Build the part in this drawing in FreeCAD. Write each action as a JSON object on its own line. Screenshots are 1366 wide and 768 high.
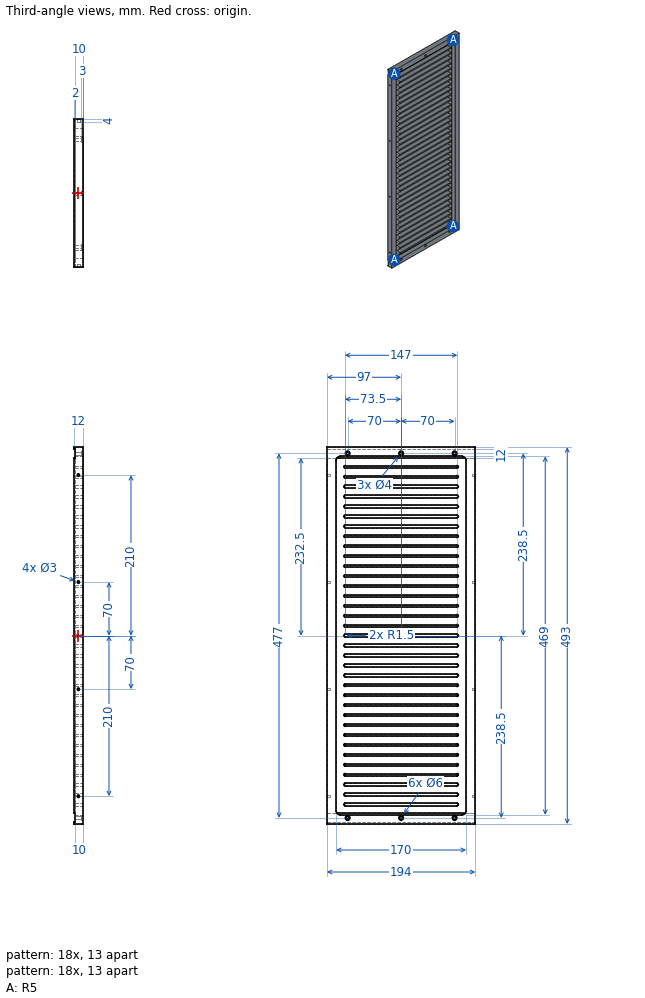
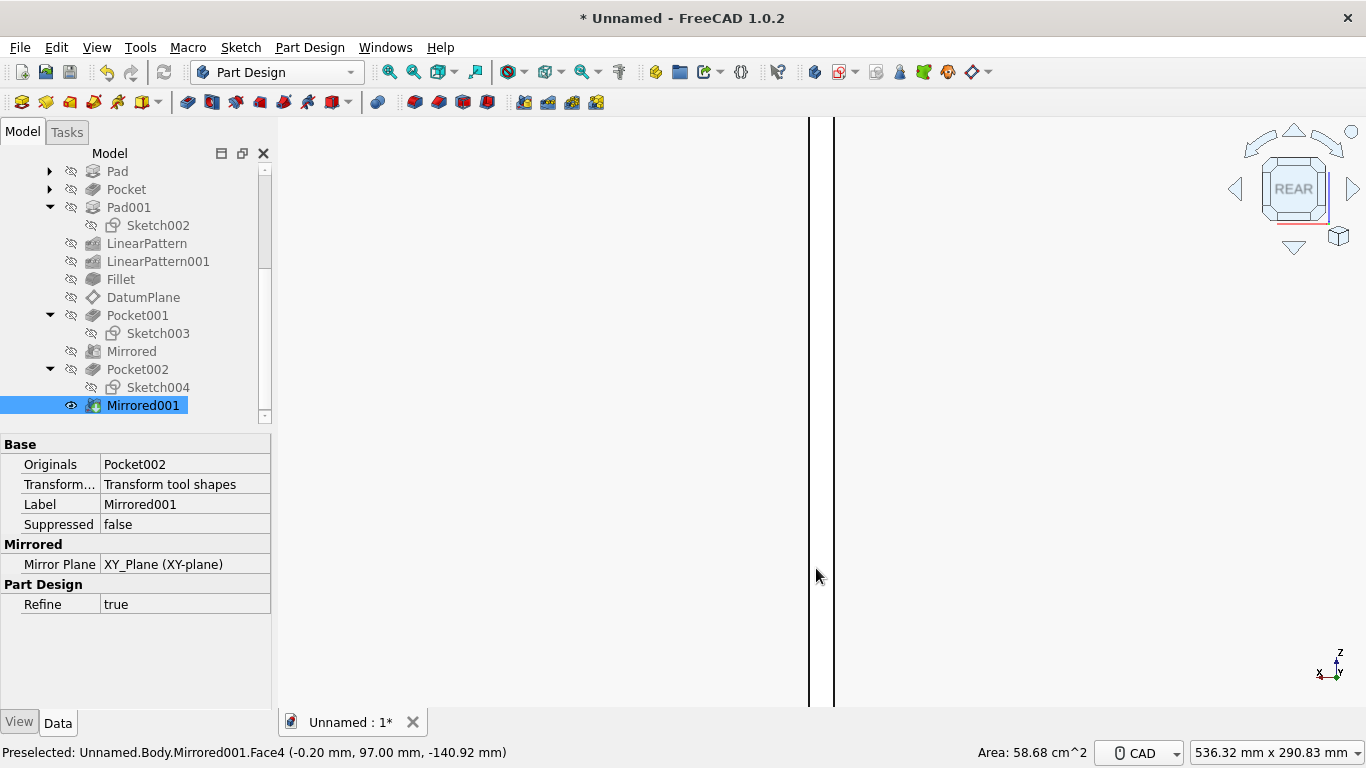
{"action": "left_click", "coordinate": [840, 72]}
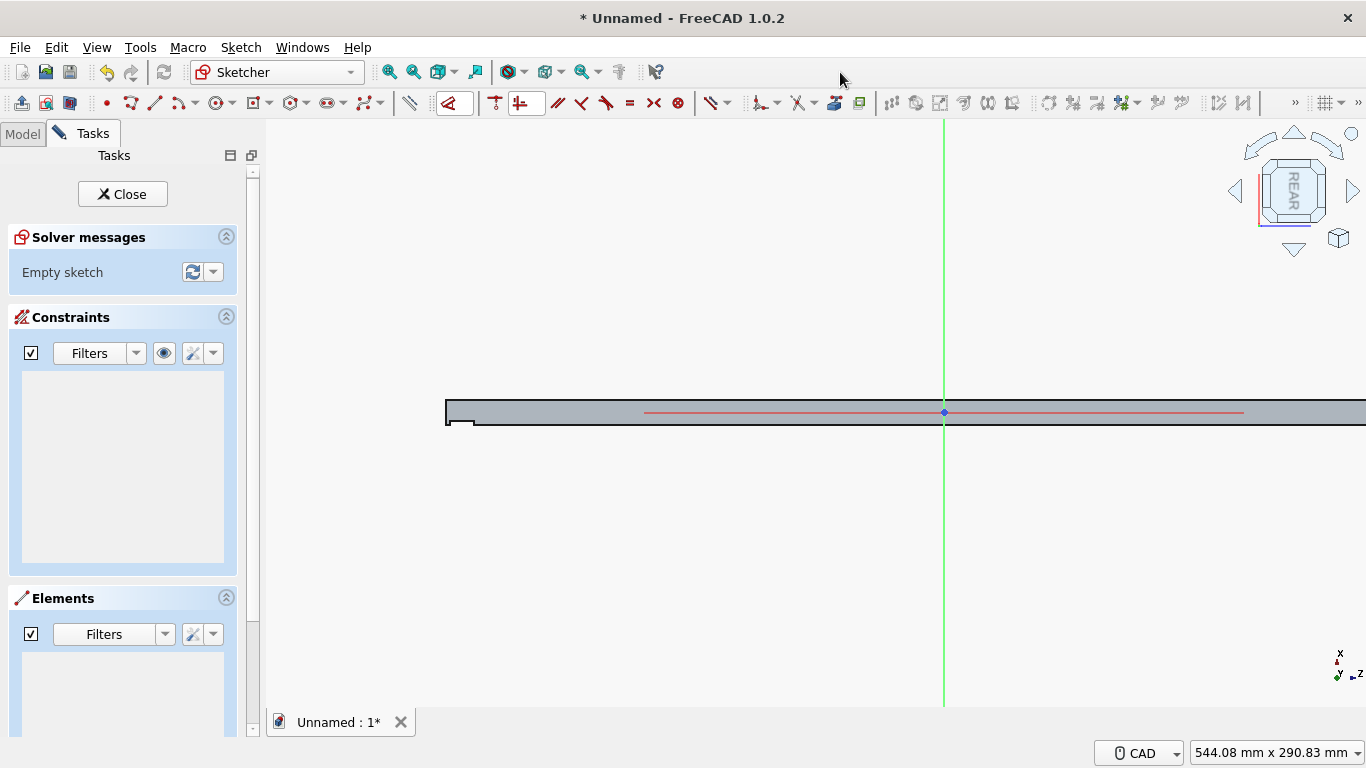
{"action": "scroll", "coordinate": [347, 414], "scroll_direction": "down", "scroll_amount": 2}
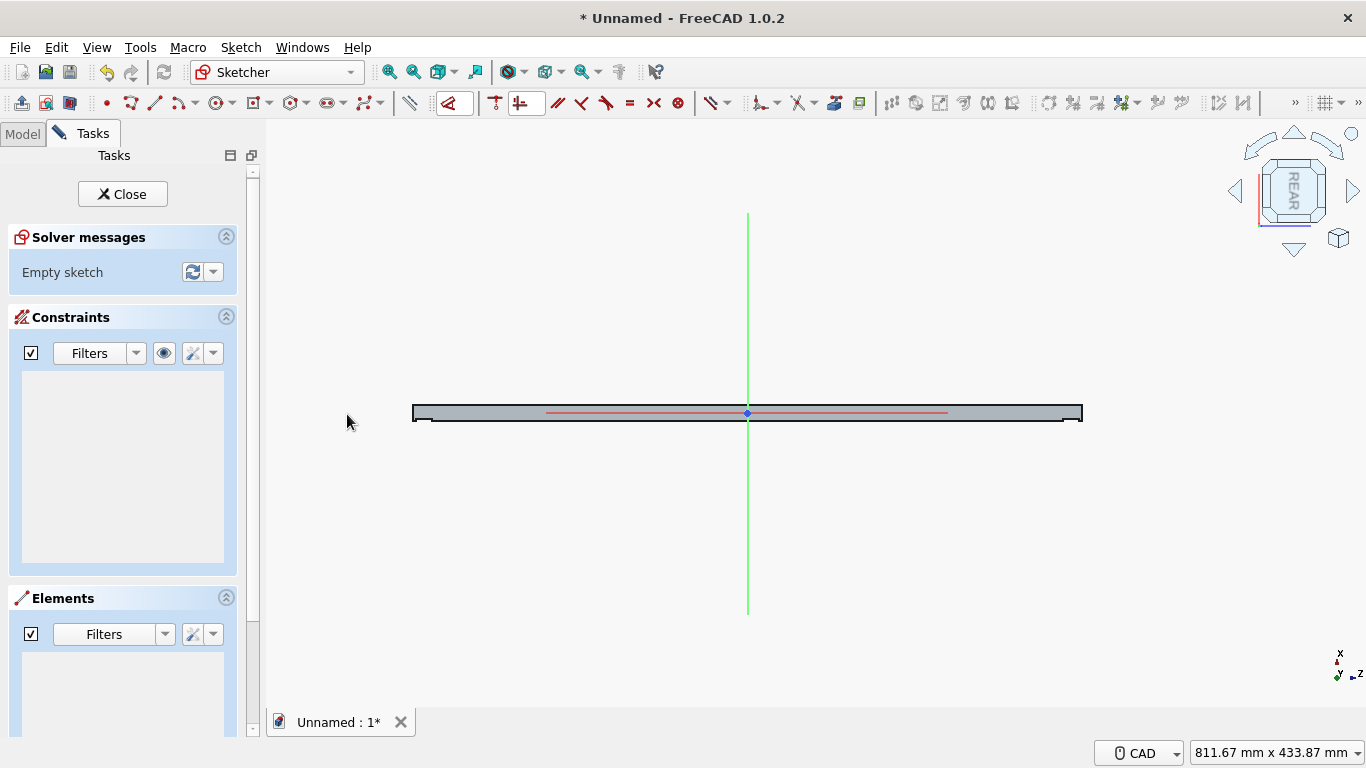
{"action": "left_click", "coordinate": [216, 104]}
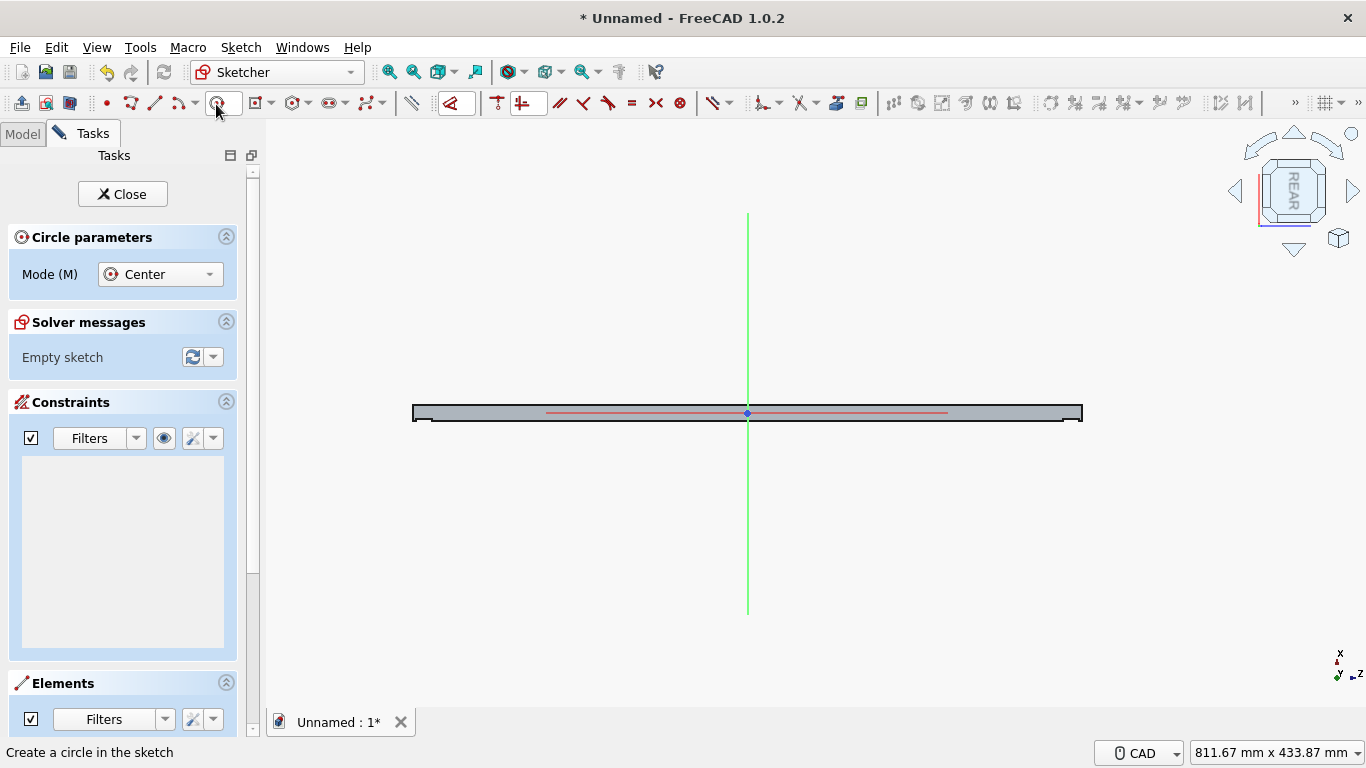
{"action": "scroll", "coordinate": [842, 413], "scroll_direction": "up", "scroll_amount": 13}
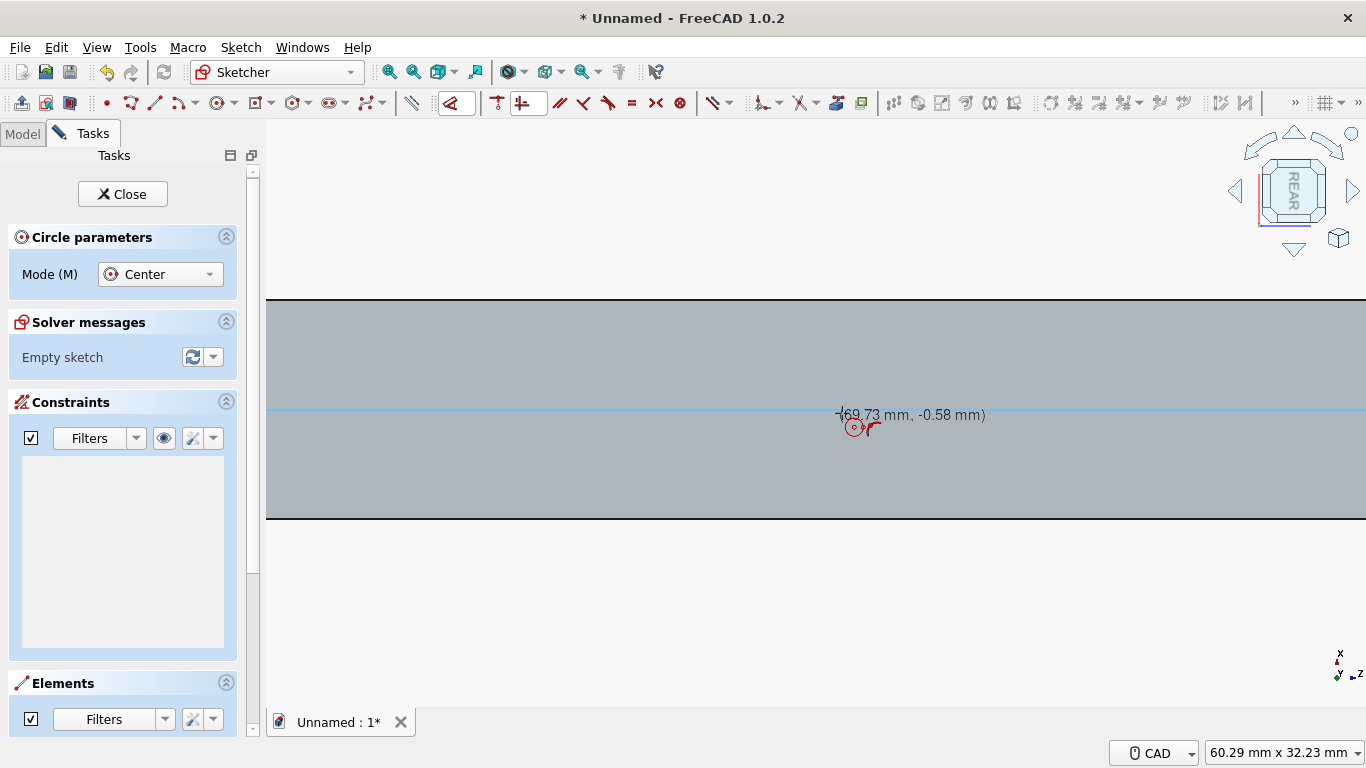
{"action": "scroll", "coordinate": [866, 413], "scroll_direction": "down", "scroll_amount": 12}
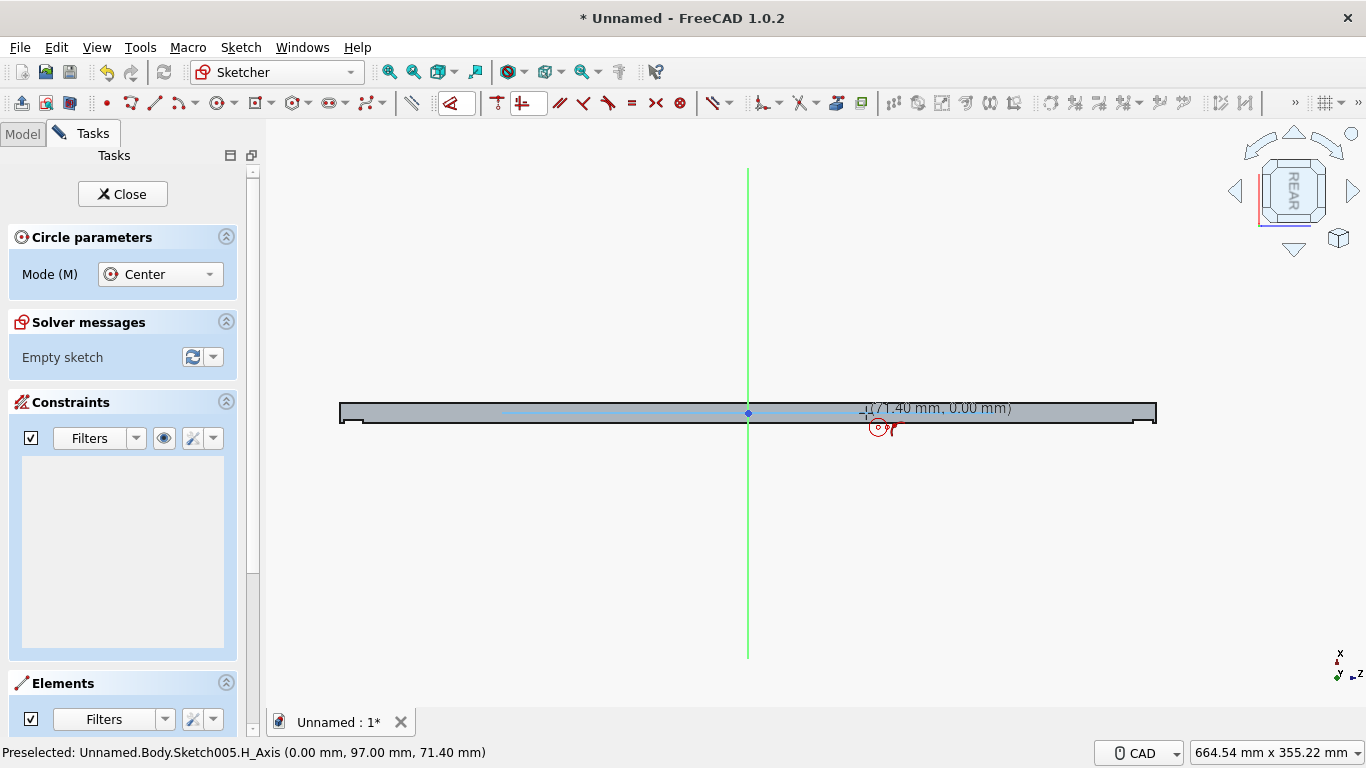
{"action": "left_click", "coordinate": [864, 413]}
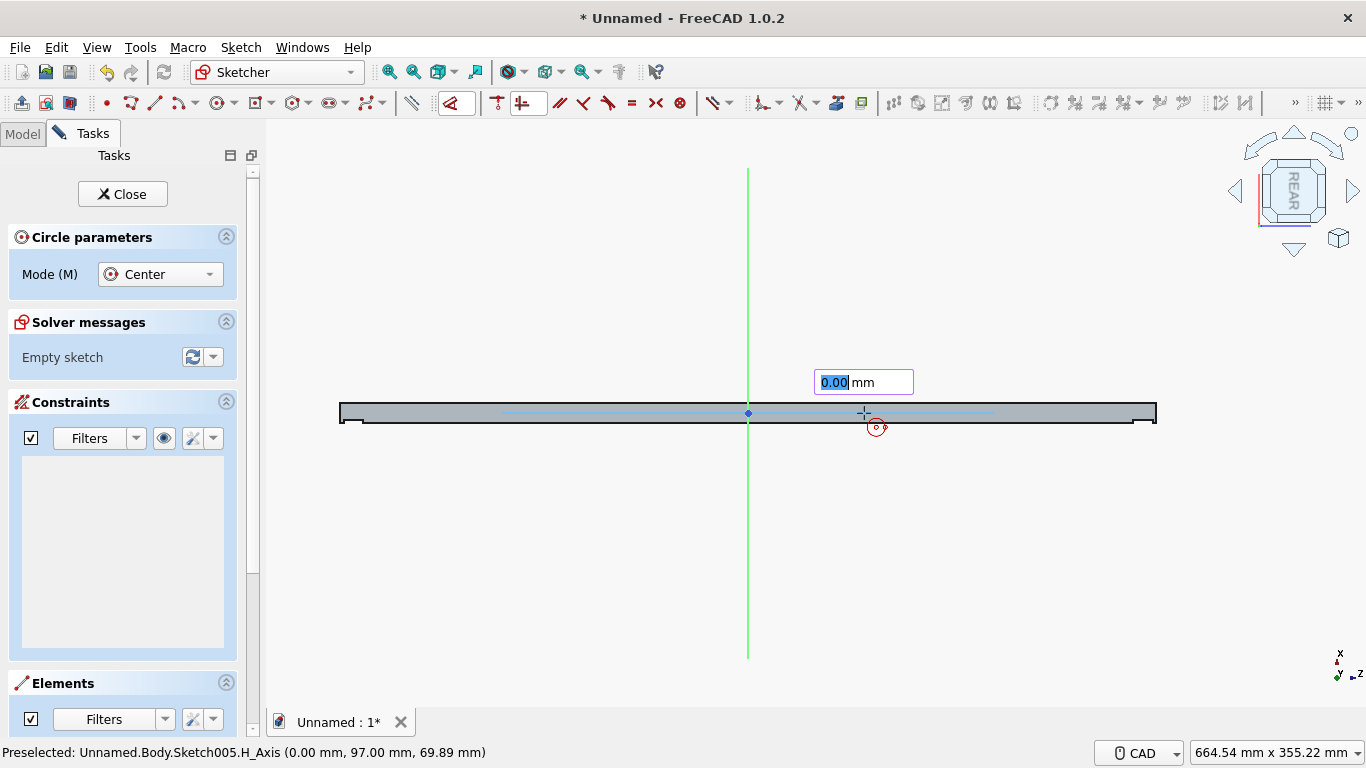
{"action": "scroll", "coordinate": [863, 415], "scroll_direction": "up", "scroll_amount": 10}
{"action": "mouse_move", "coordinate": [862, 415]}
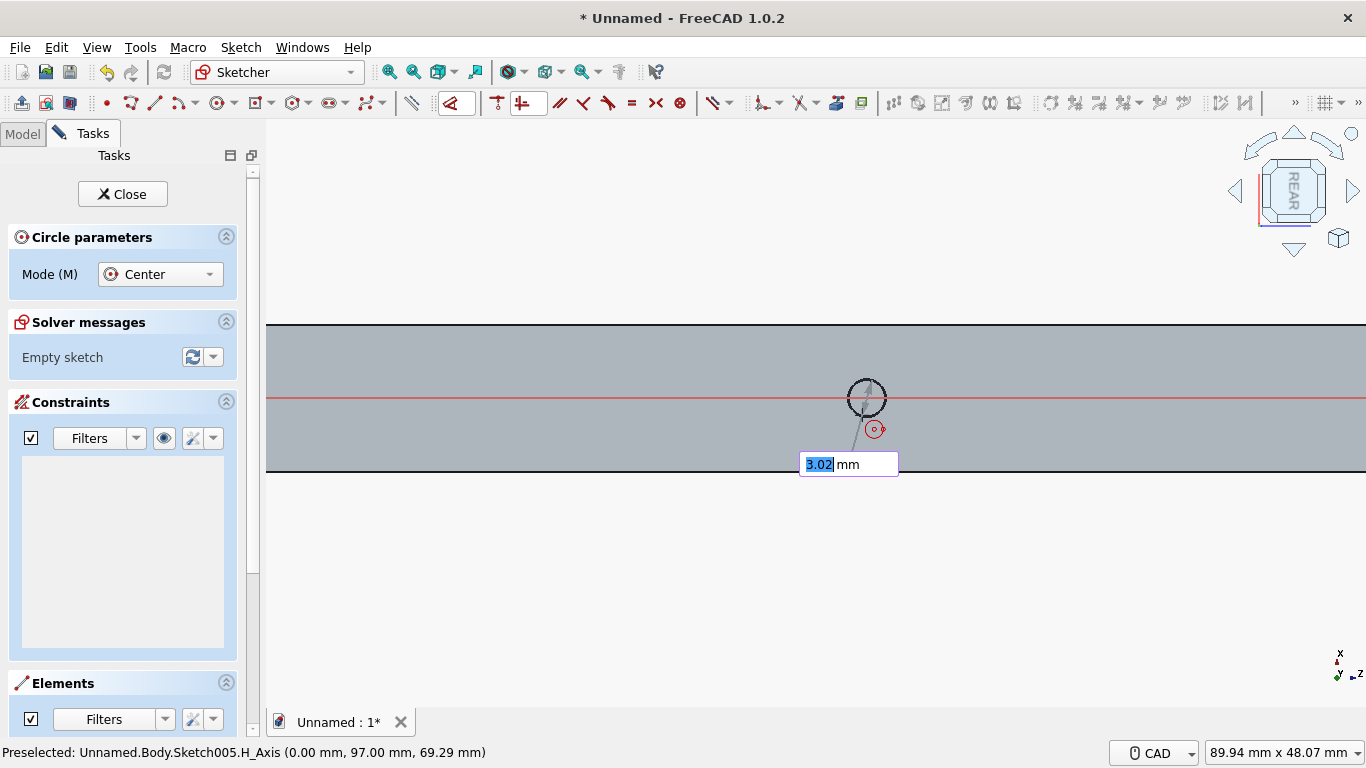
{"action": "type", "text": "3"}
{"action": "key", "text": "Return"}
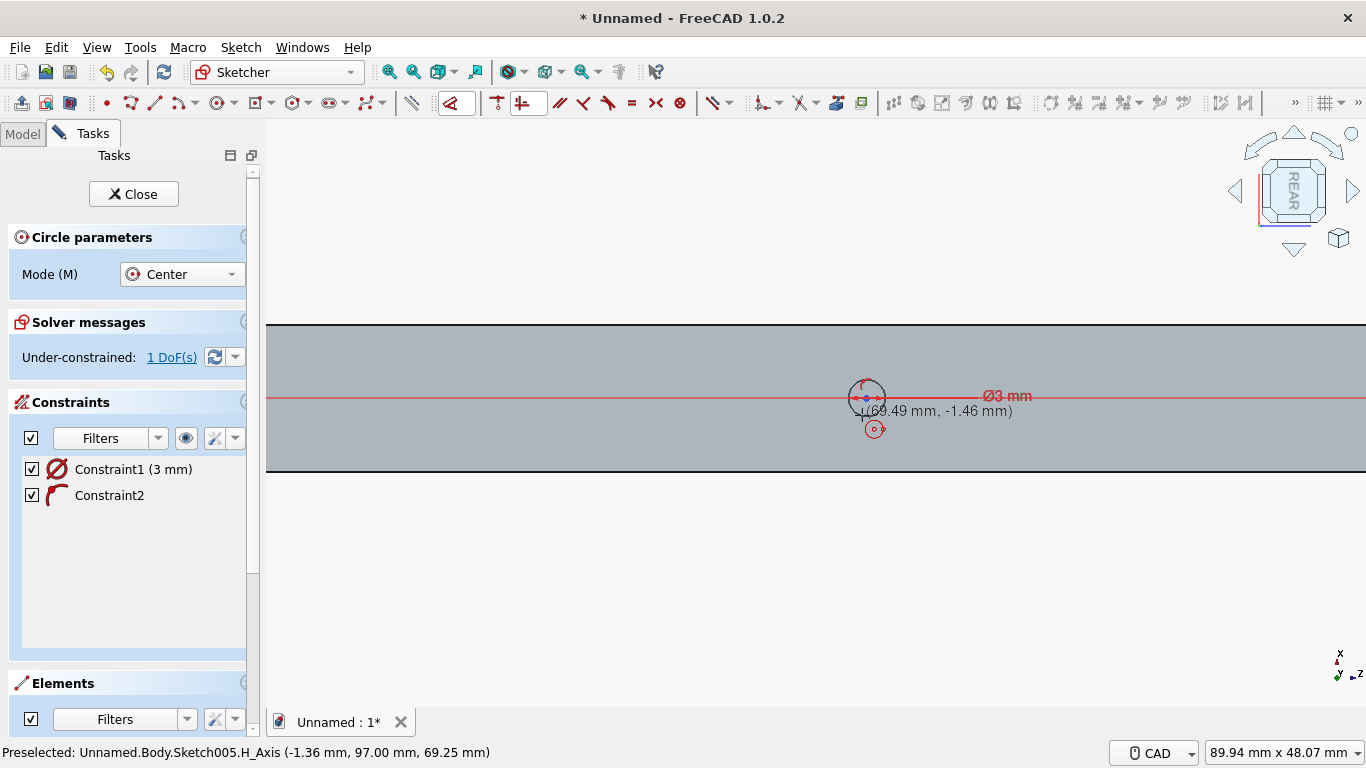
{"action": "scroll", "coordinate": [863, 415], "scroll_direction": "down", "scroll_amount": 10}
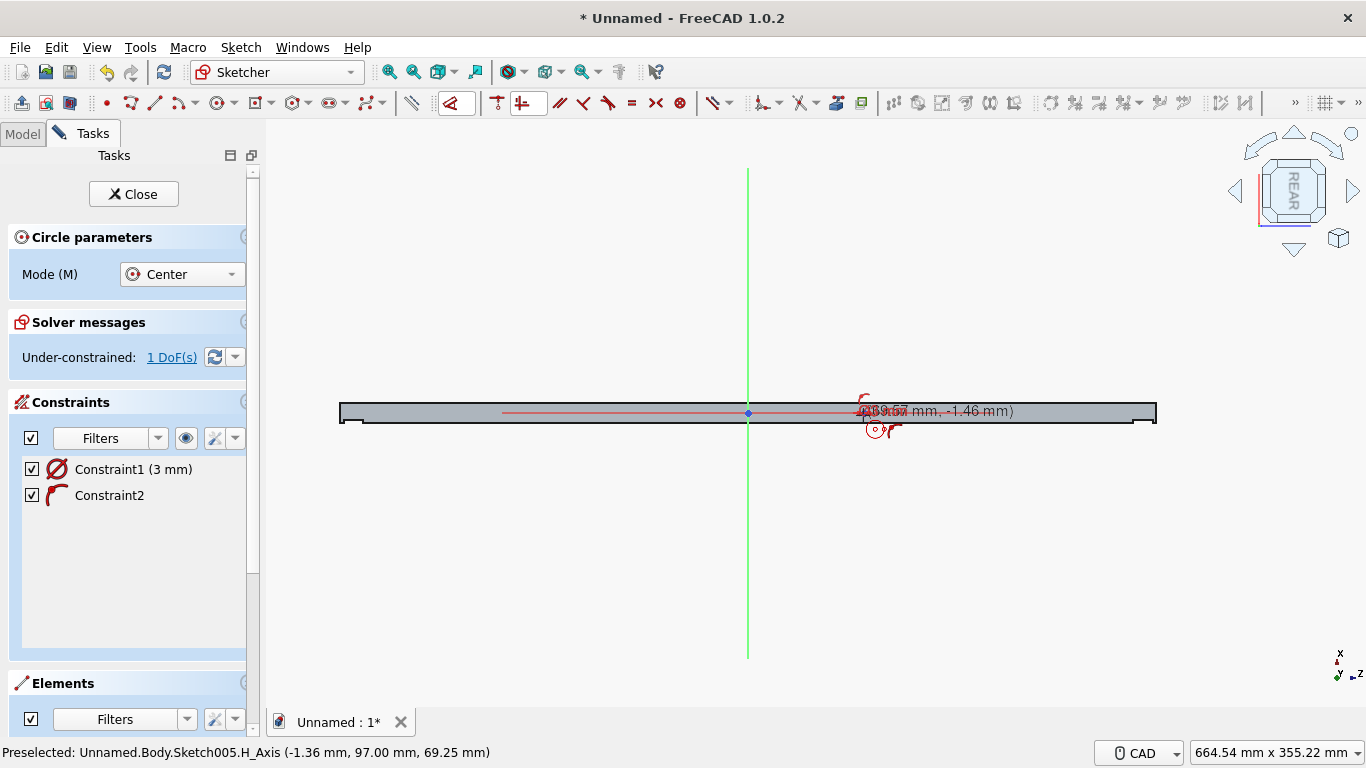
{"action": "scroll", "coordinate": [1096, 413], "scroll_direction": "up", "scroll_amount": 12}